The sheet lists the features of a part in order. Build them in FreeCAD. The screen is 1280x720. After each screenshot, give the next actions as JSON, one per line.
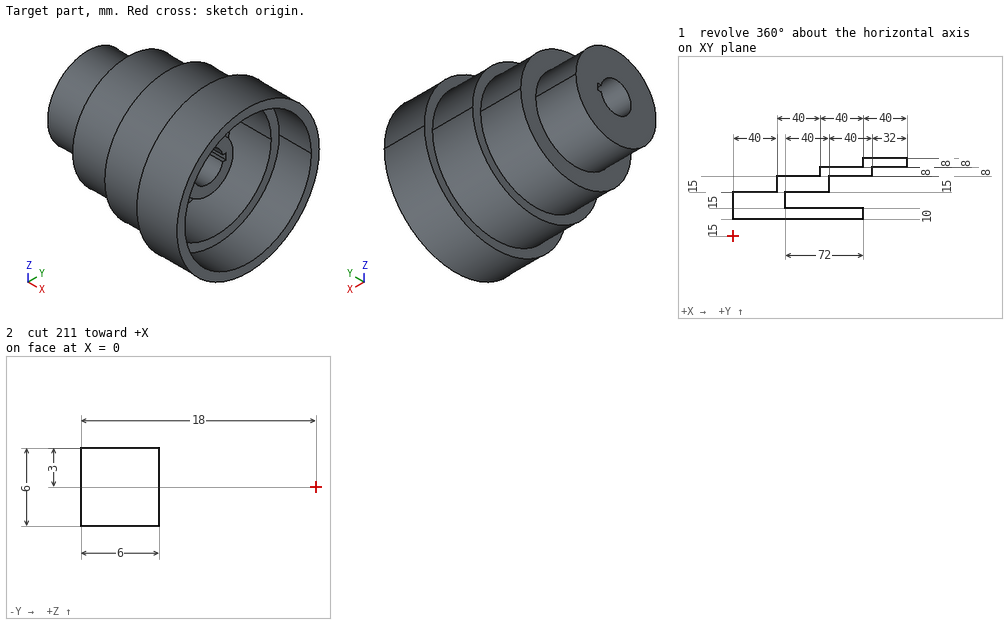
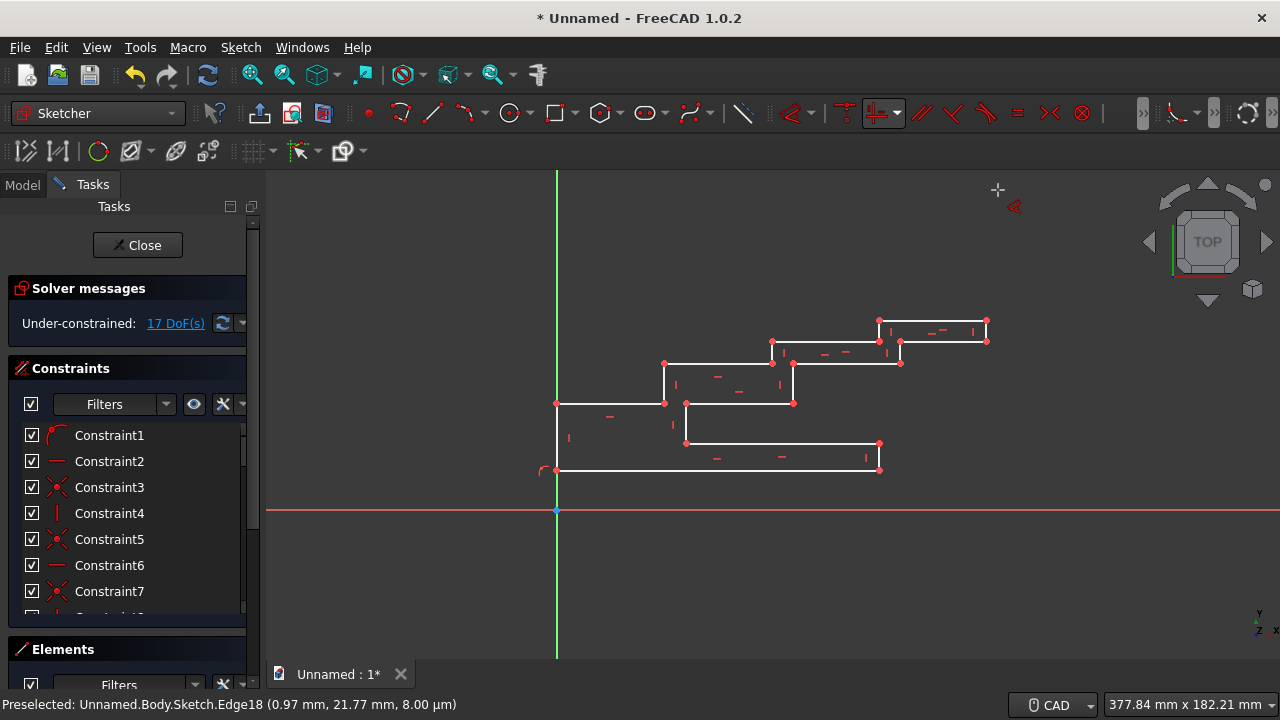
{"action": "scroll", "coordinate": [900, 353], "scroll_direction": "up", "scroll_amount": 4}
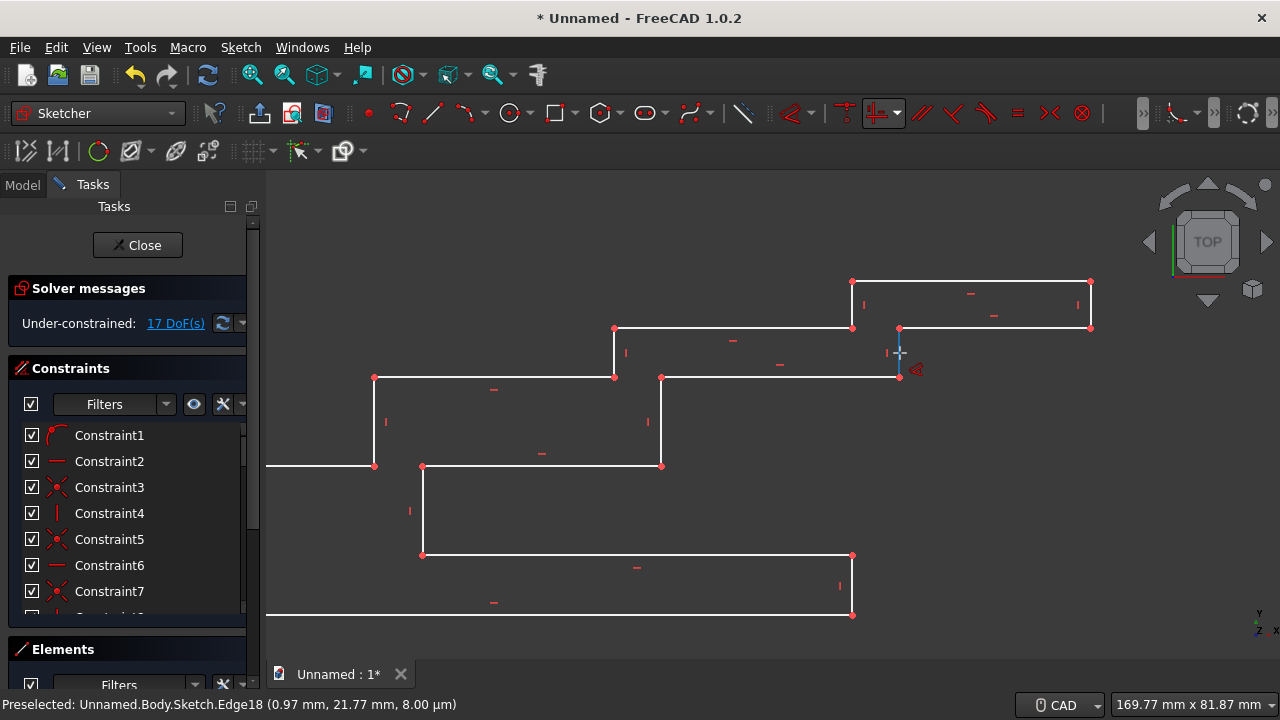
{"action": "left_click", "coordinate": [899, 353]}
{"action": "left_click", "coordinate": [933, 353]}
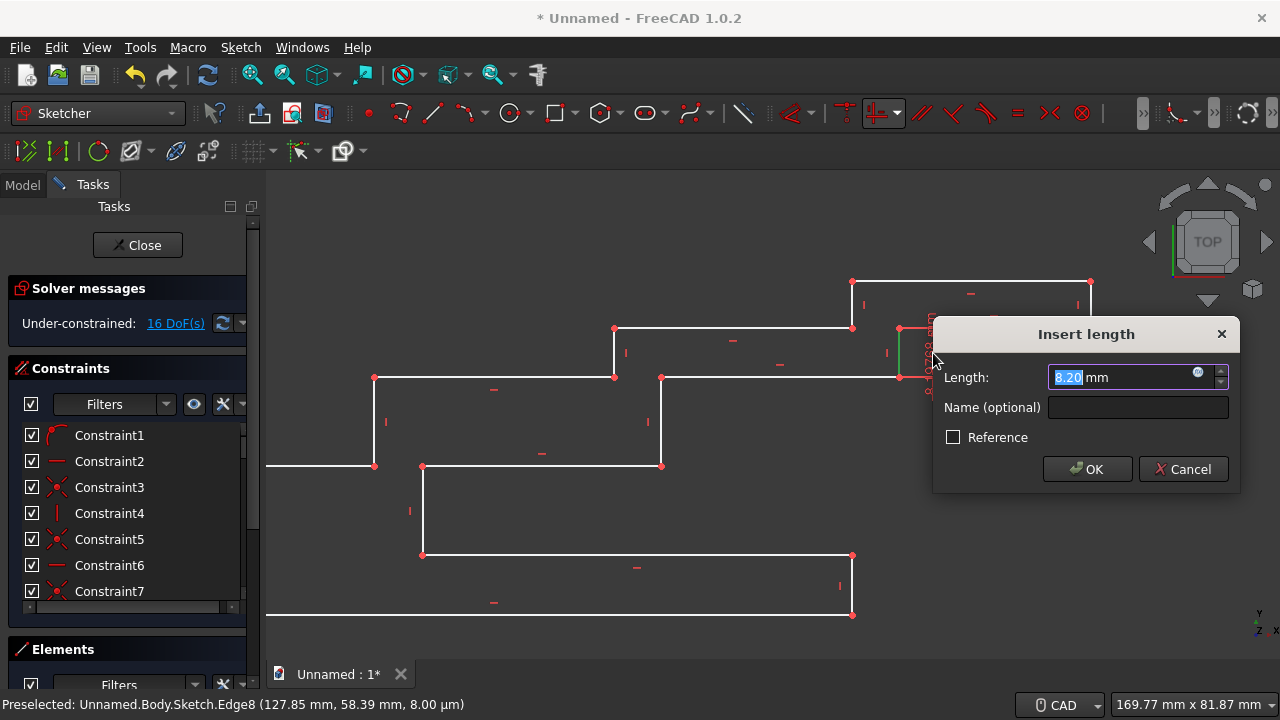
{"action": "type", "text": "8"}
{"action": "key", "text": "Return"}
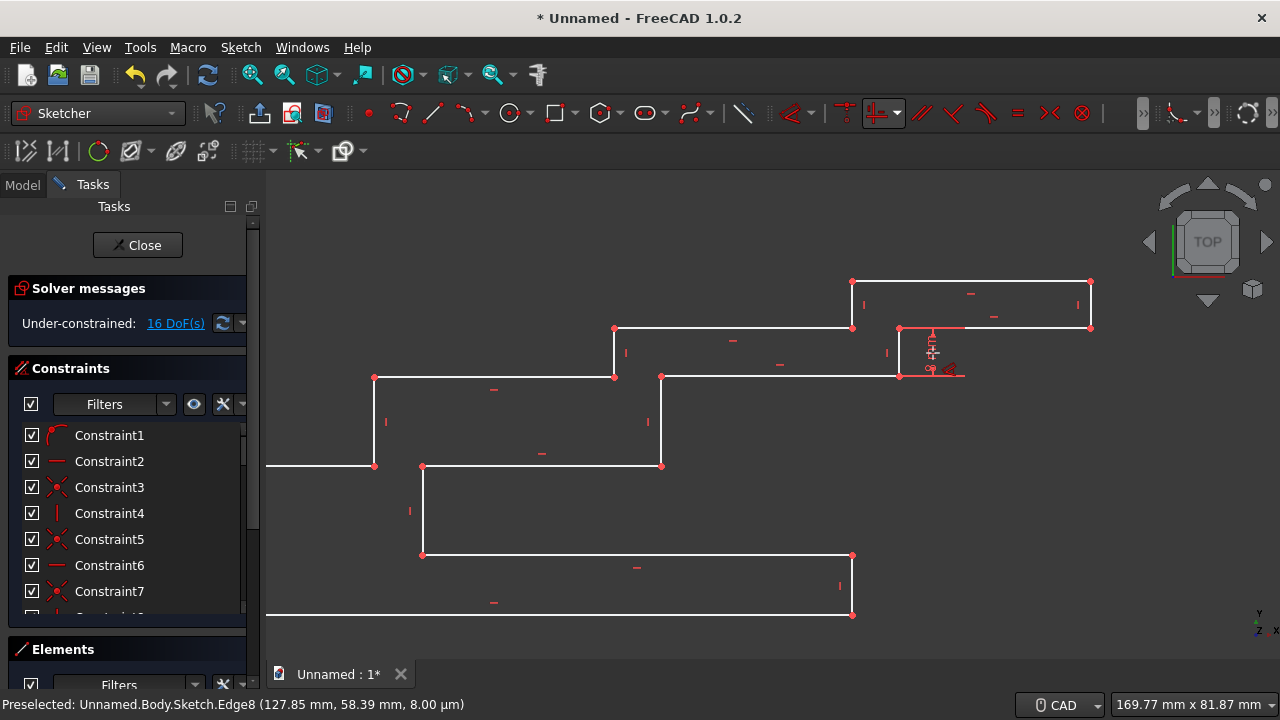
{"action": "left_click", "coordinate": [1091, 314]}
{"action": "left_click", "coordinate": [1057, 305]}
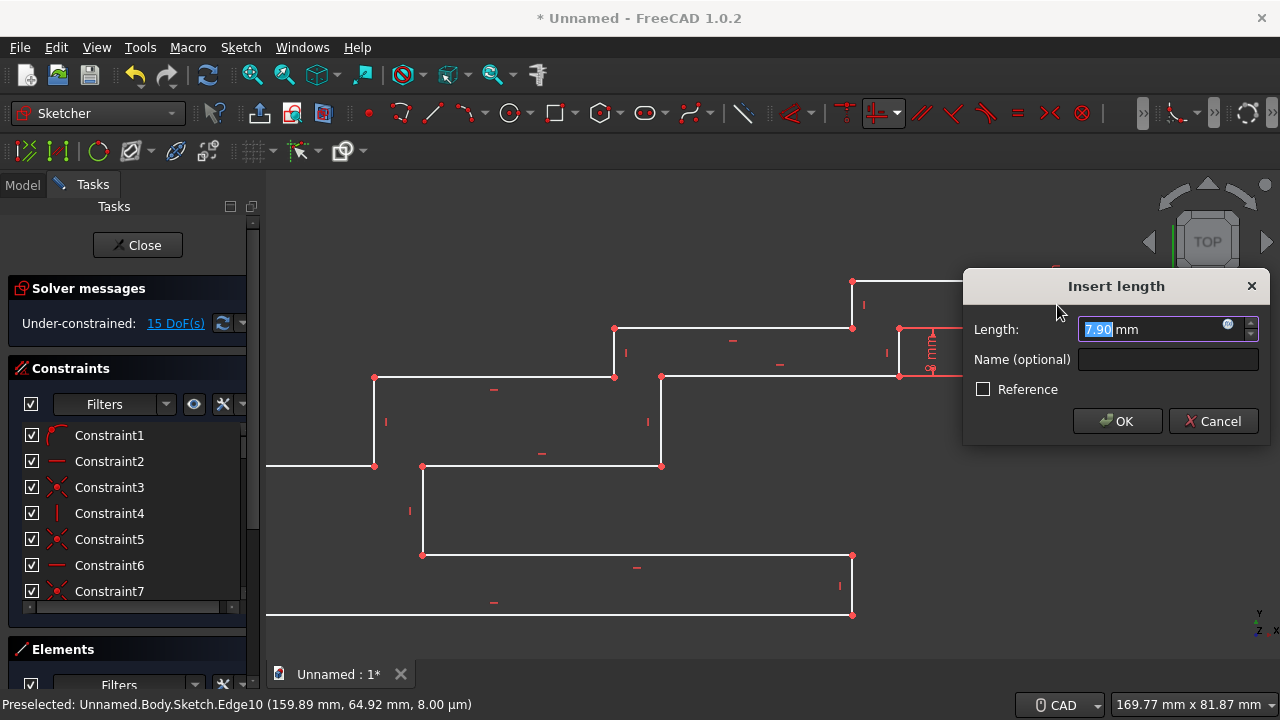
{"action": "type", "text": "8"}
{"action": "key", "text": "Return"}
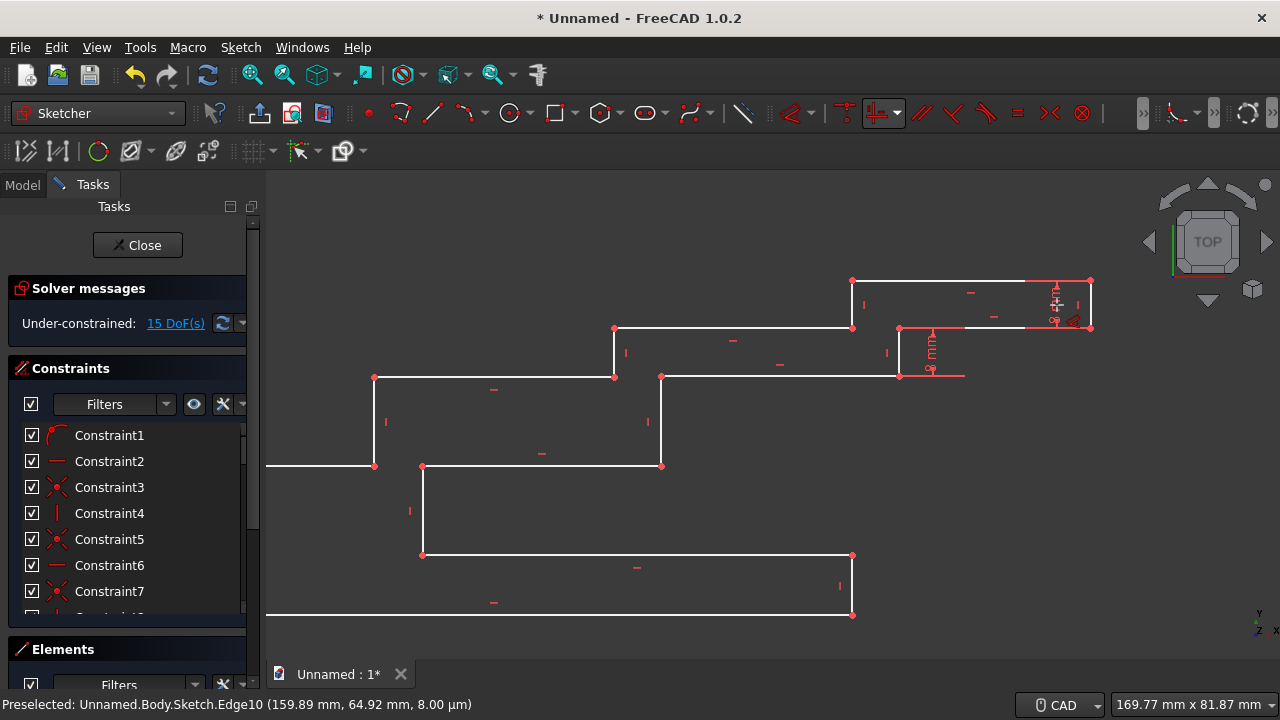
{"action": "left_click", "coordinate": [852, 295]}
{"action": "left_click", "coordinate": [886, 304]}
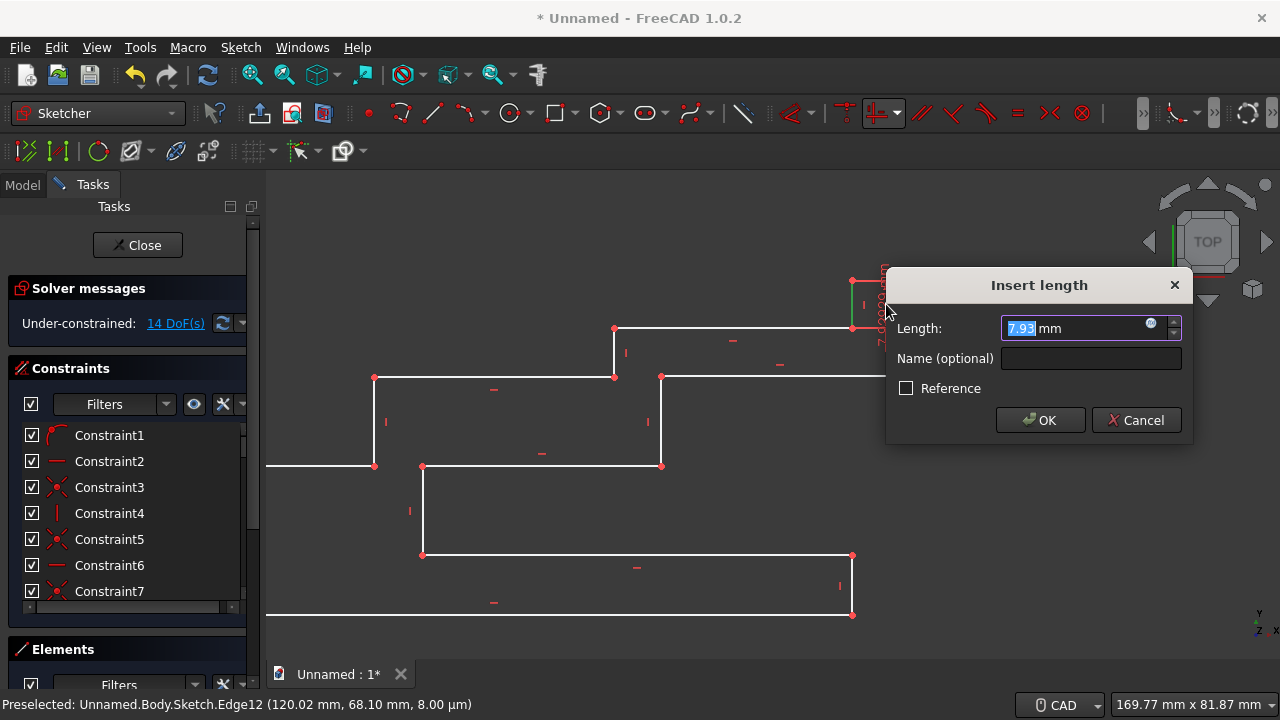
{"action": "type", "text": "8"}
{"action": "key", "text": "Return"}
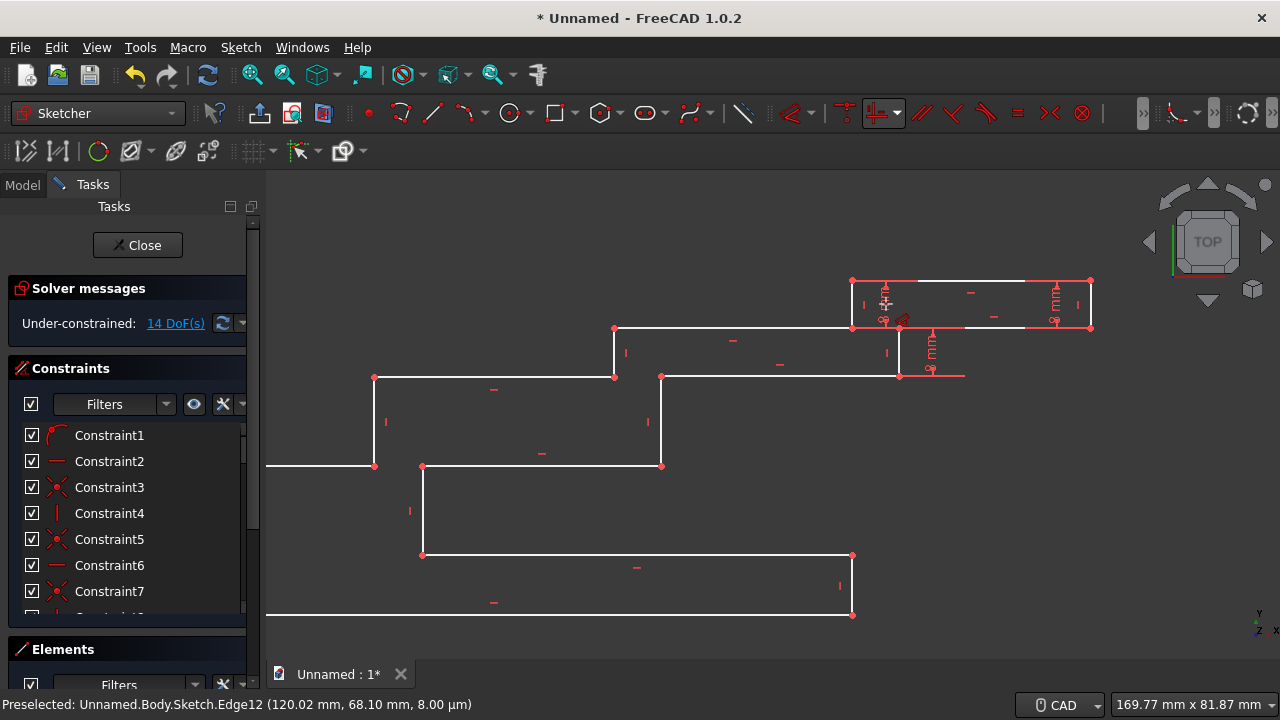
{"action": "left_click", "coordinate": [614, 343]}
{"action": "left_click", "coordinate": [648, 353]}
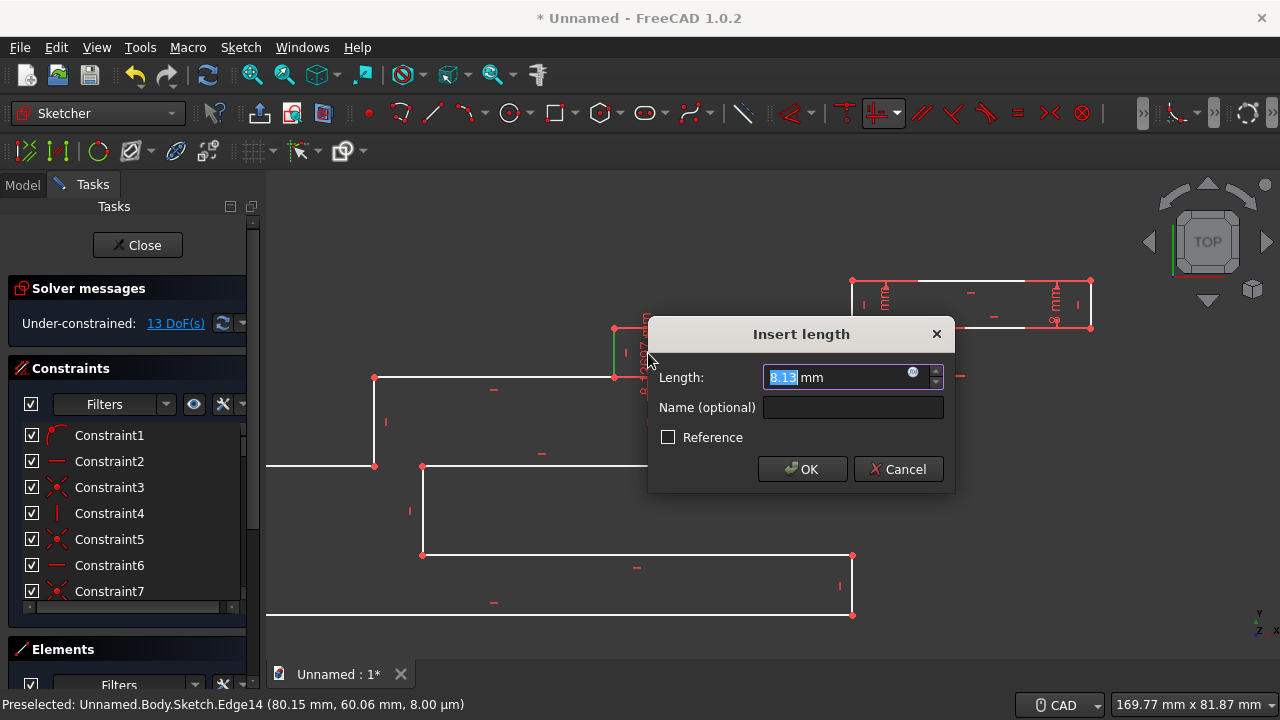
{"action": "type", "text": "8"}
{"action": "key", "text": "Return"}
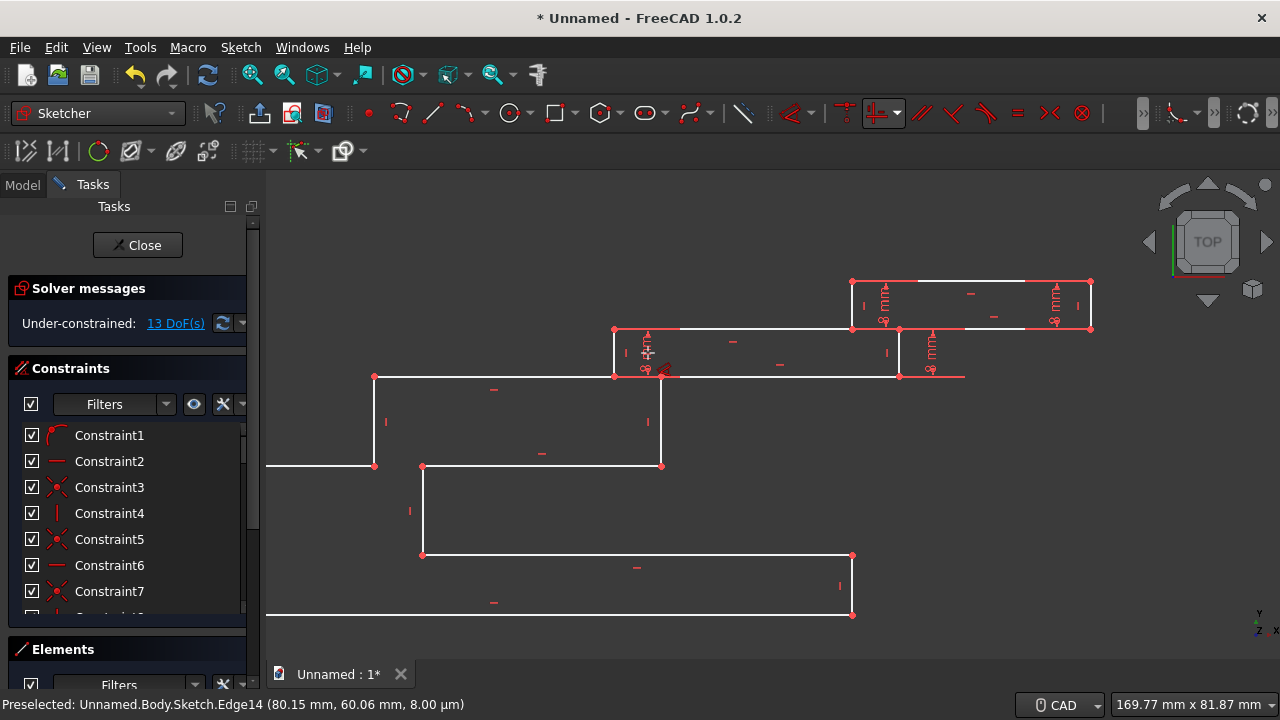
{"action": "left_click", "coordinate": [852, 597]}
{"action": "left_click", "coordinate": [886, 585]}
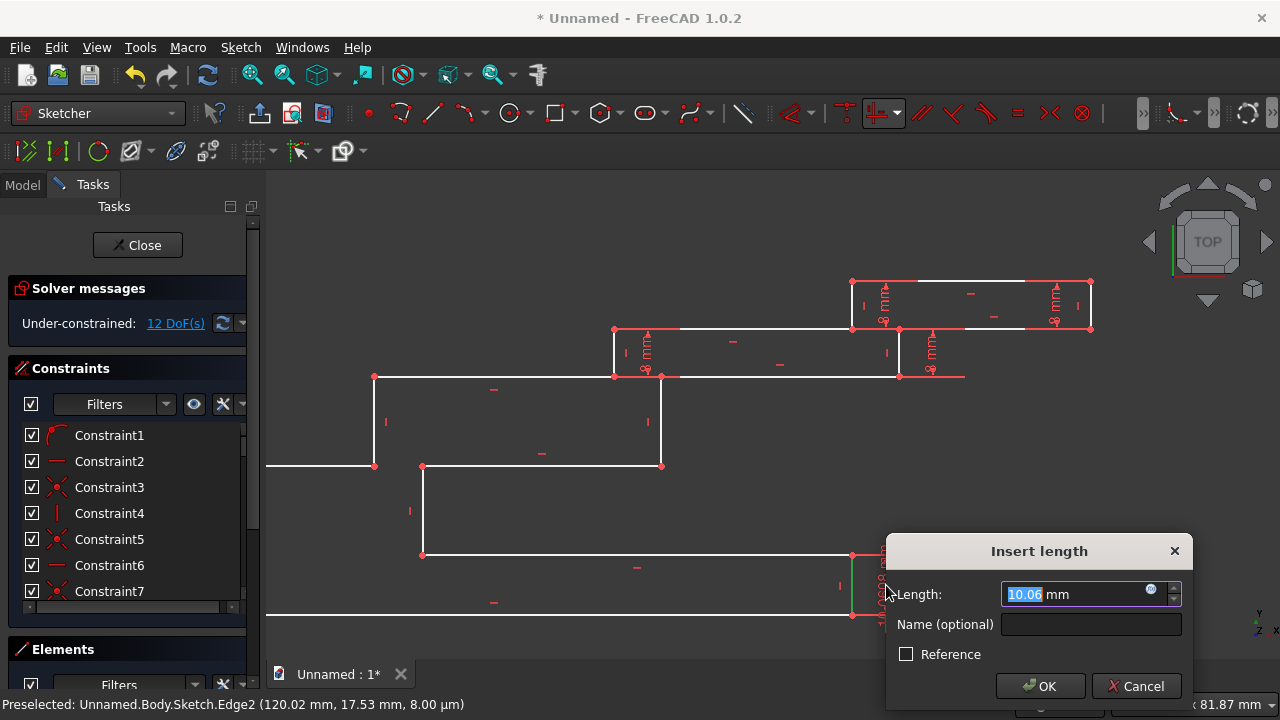
{"action": "type", "text": "10"}
{"action": "key", "text": "Return"}